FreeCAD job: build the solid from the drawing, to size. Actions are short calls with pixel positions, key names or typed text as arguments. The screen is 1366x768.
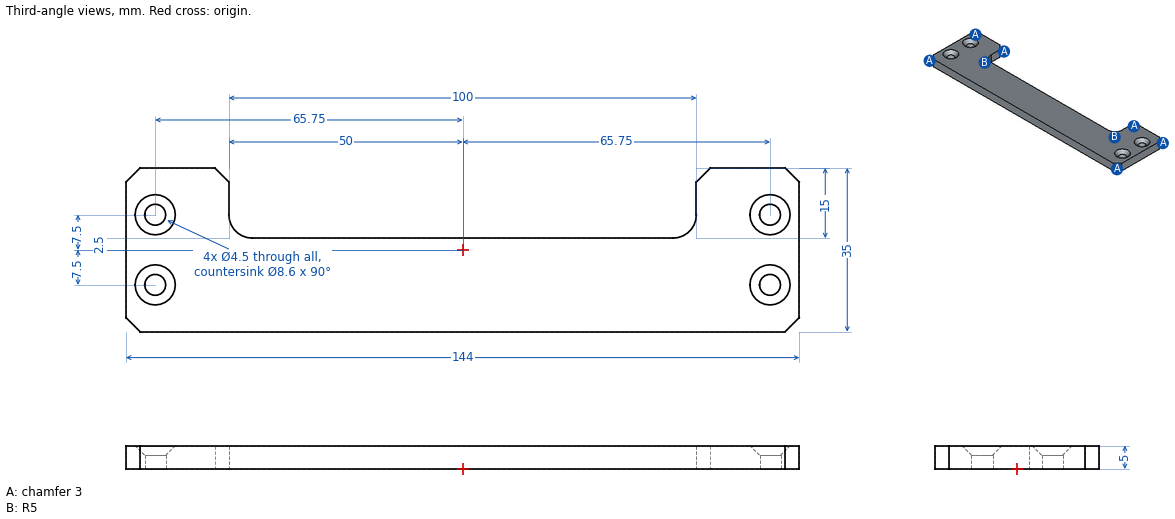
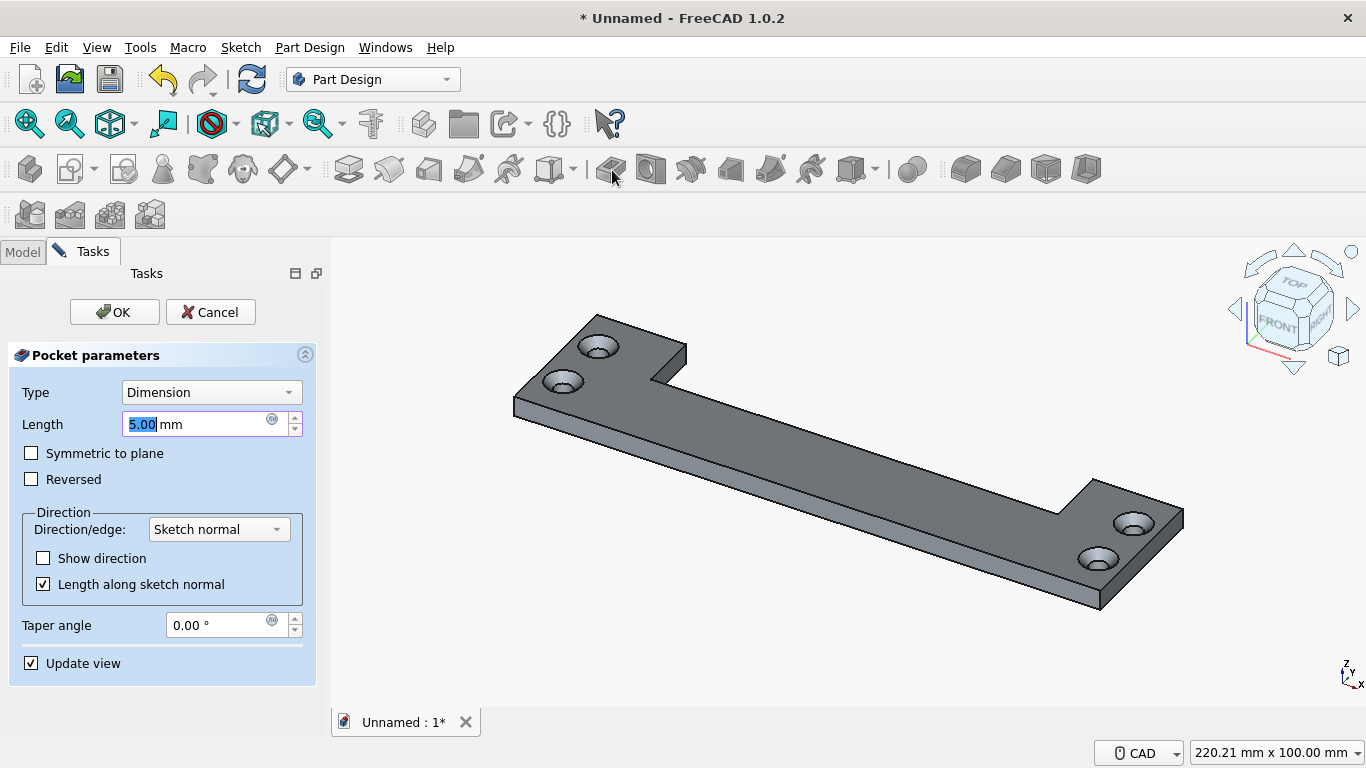
click(212, 392)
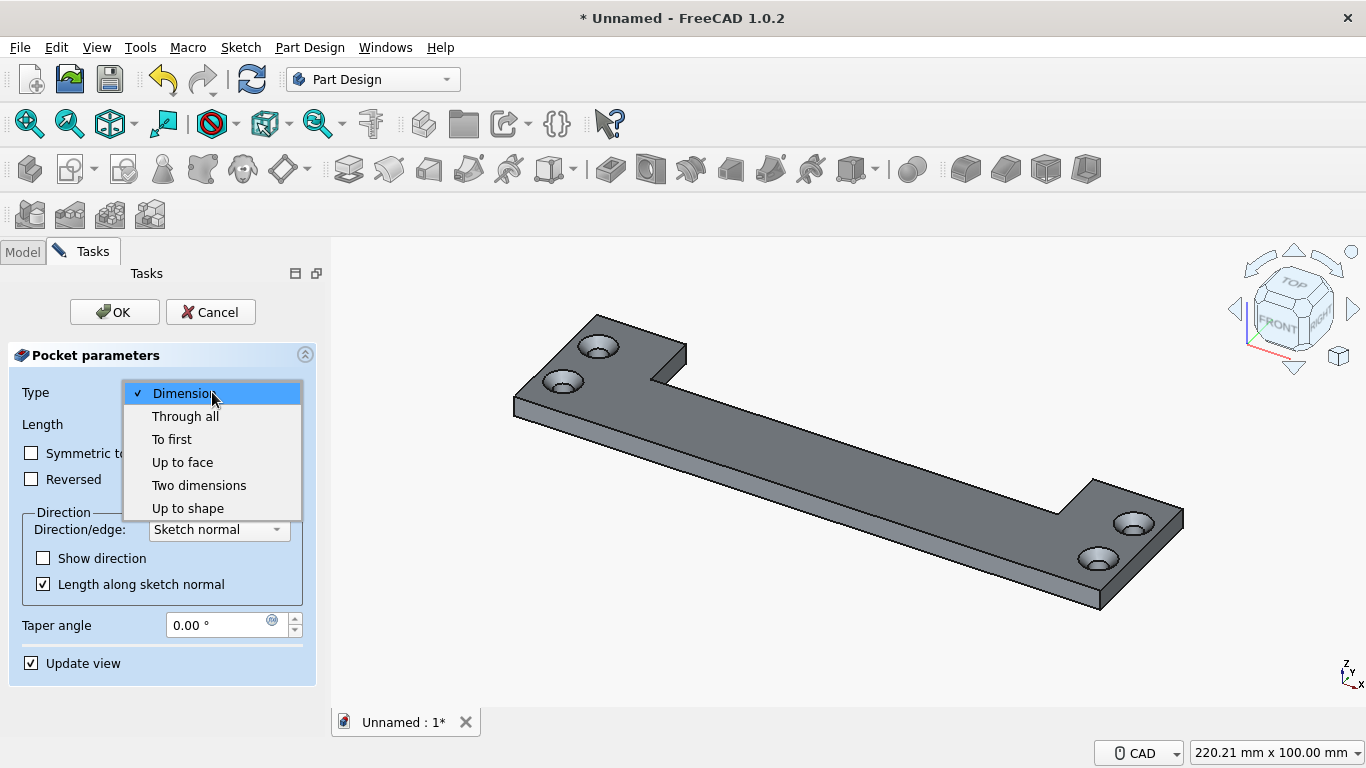
click(212, 416)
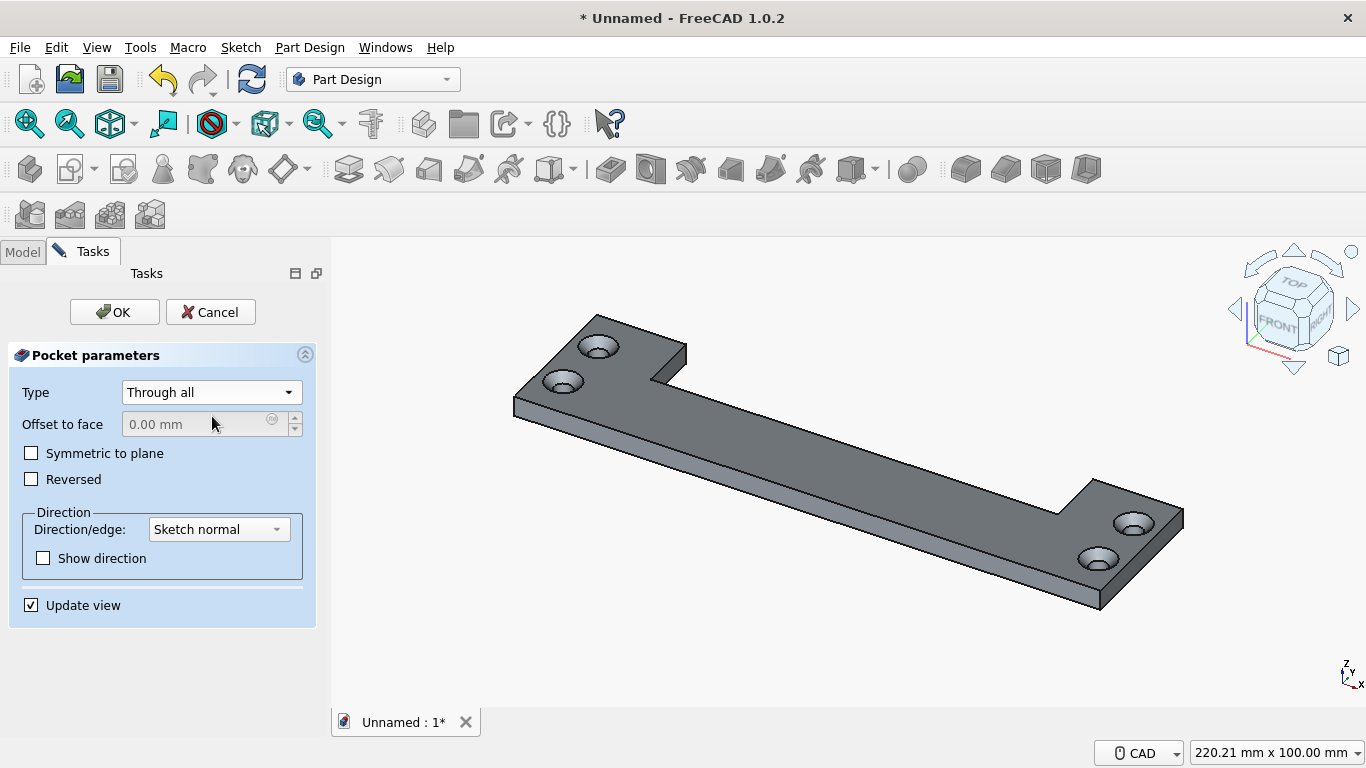
click(115, 312)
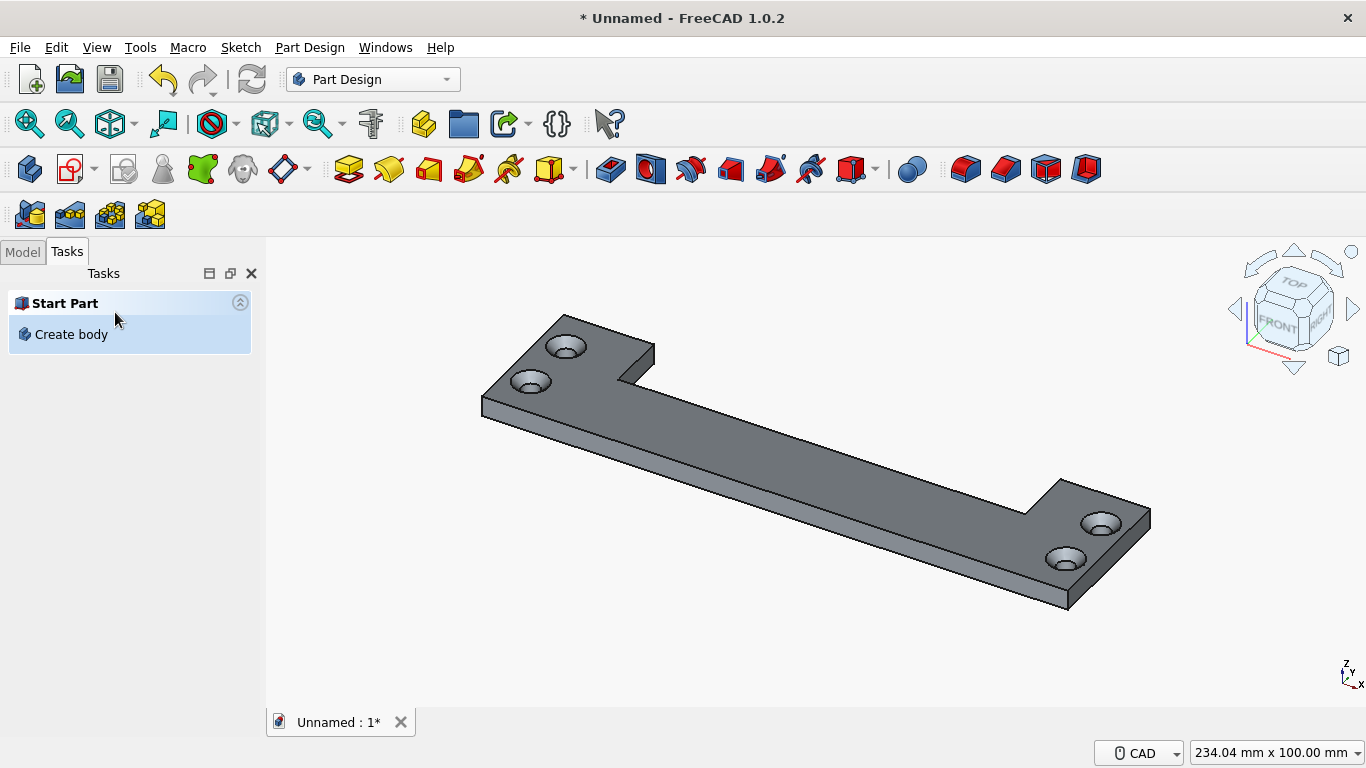
click(1068, 599)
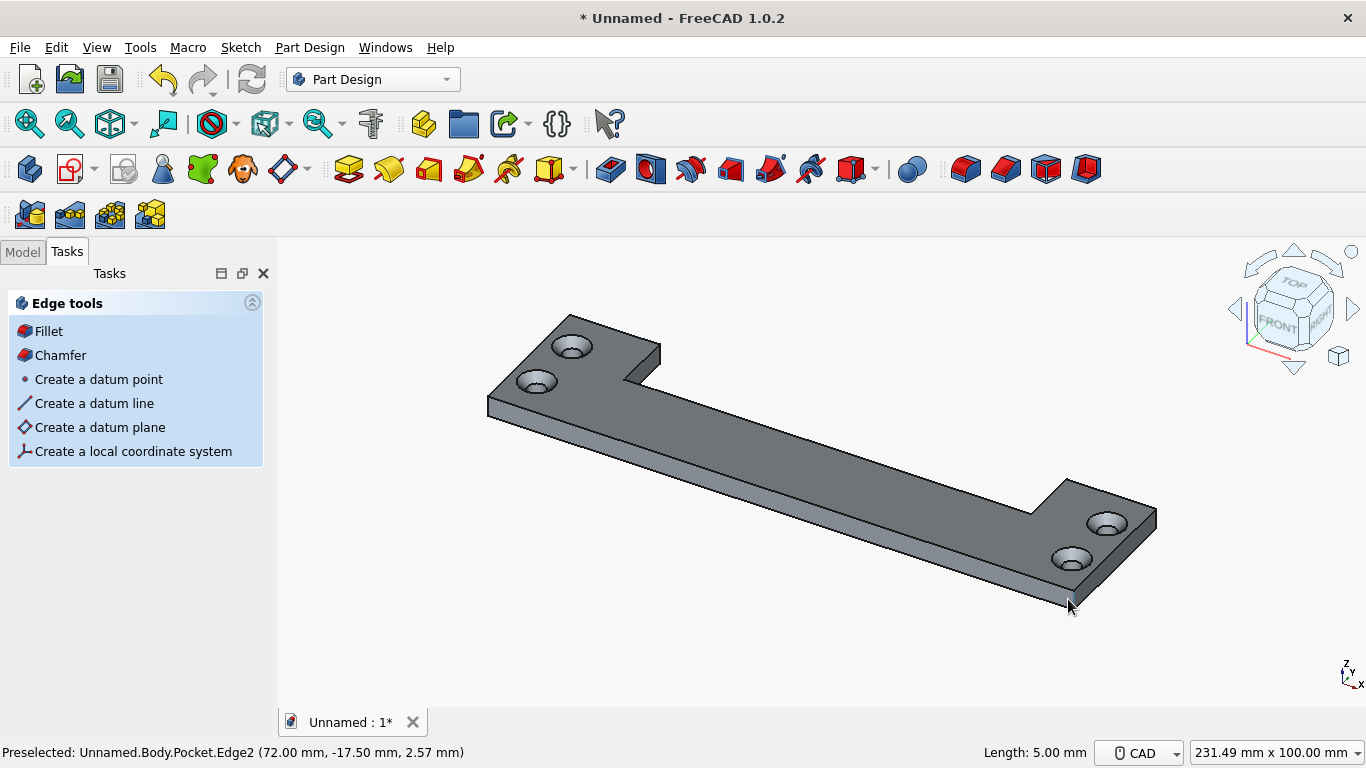
key(0)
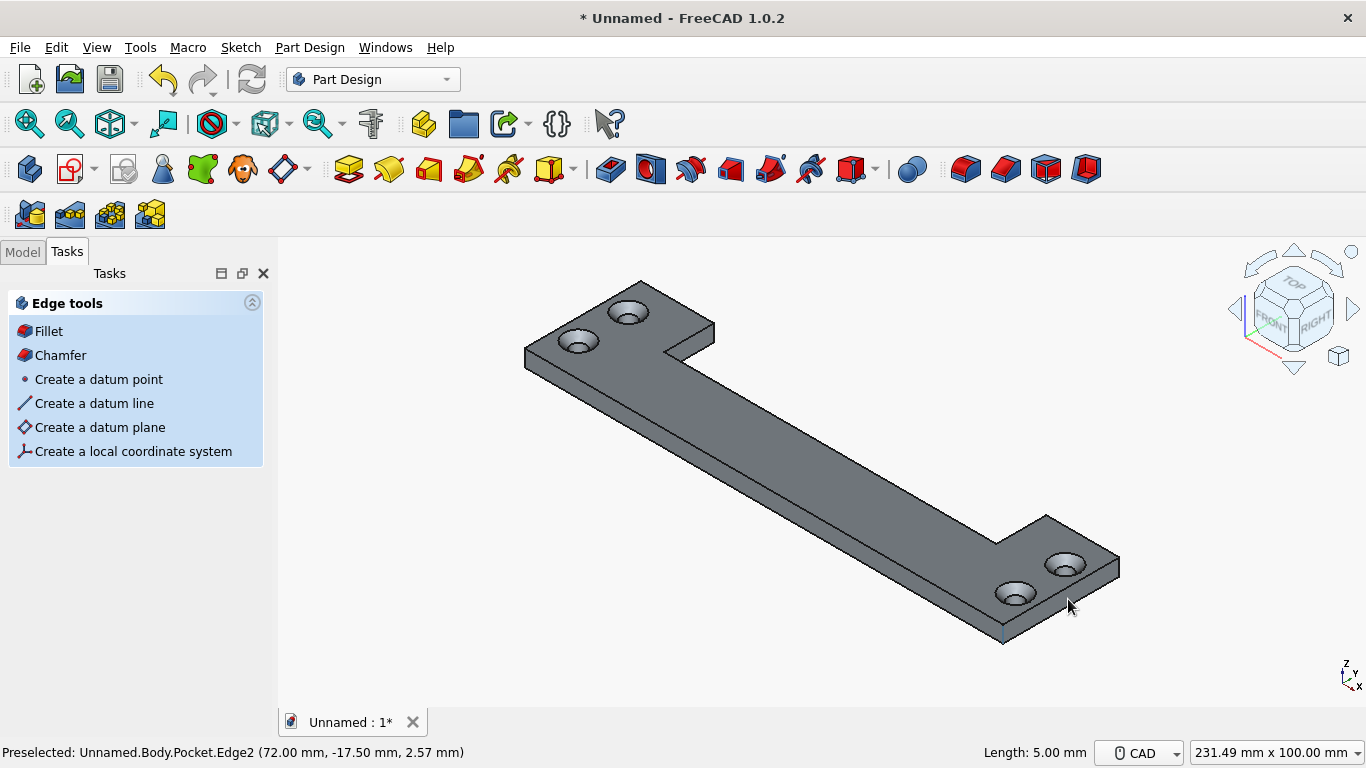
key(2)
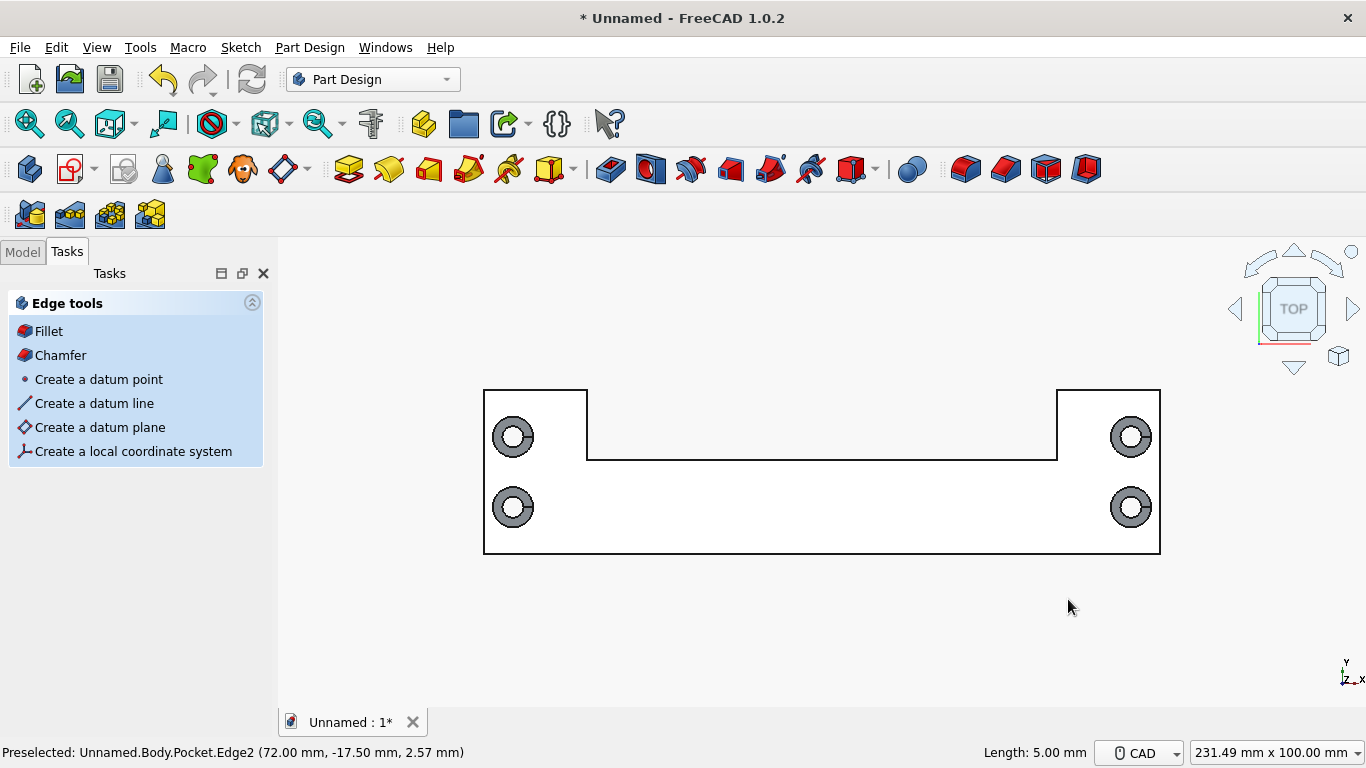
key(1)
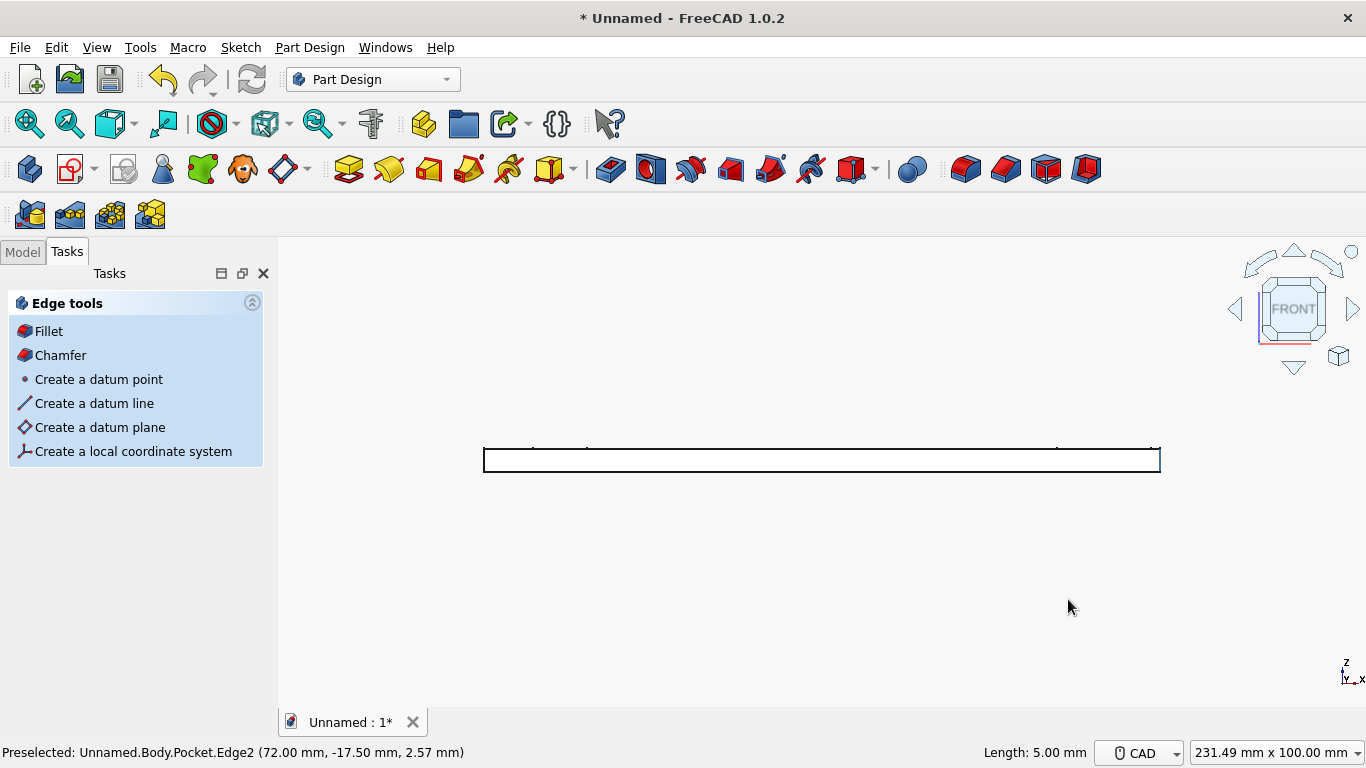
click(484, 459, ctrl)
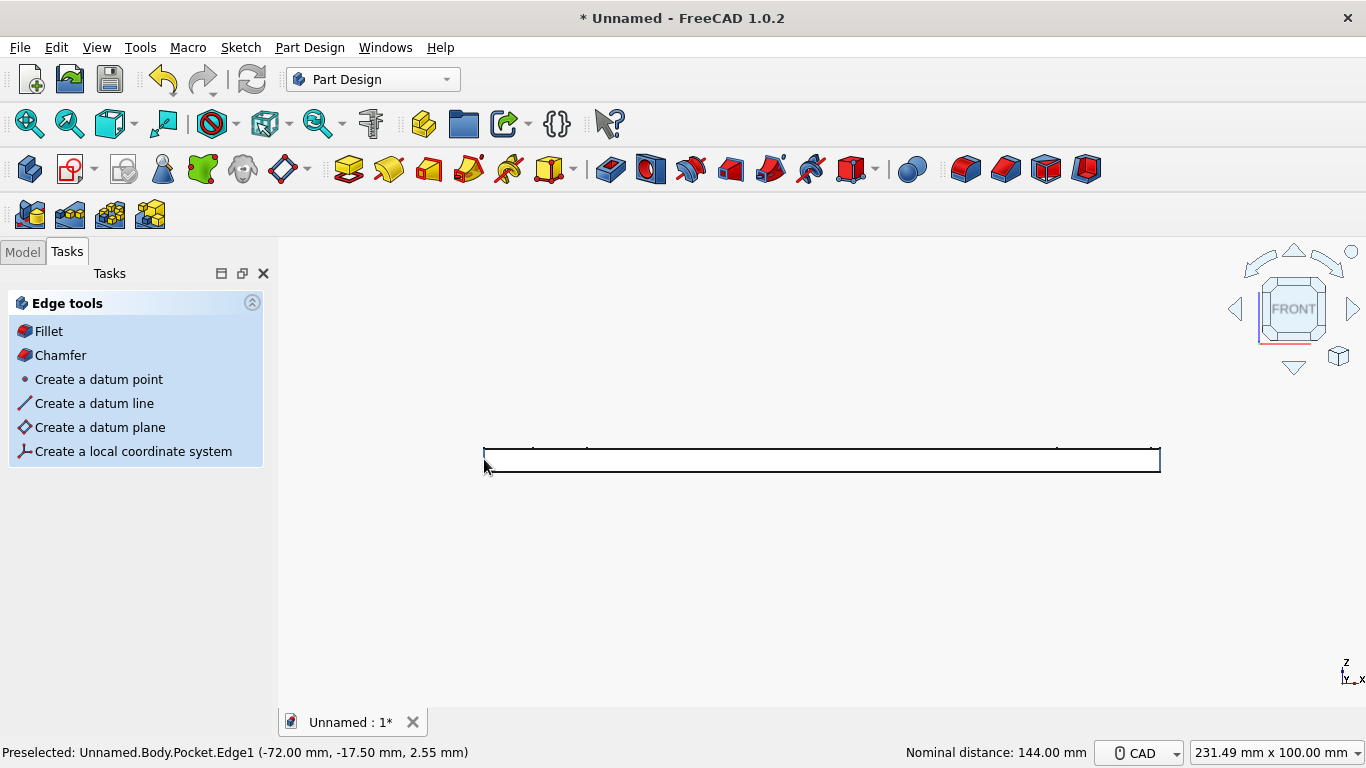
key(3)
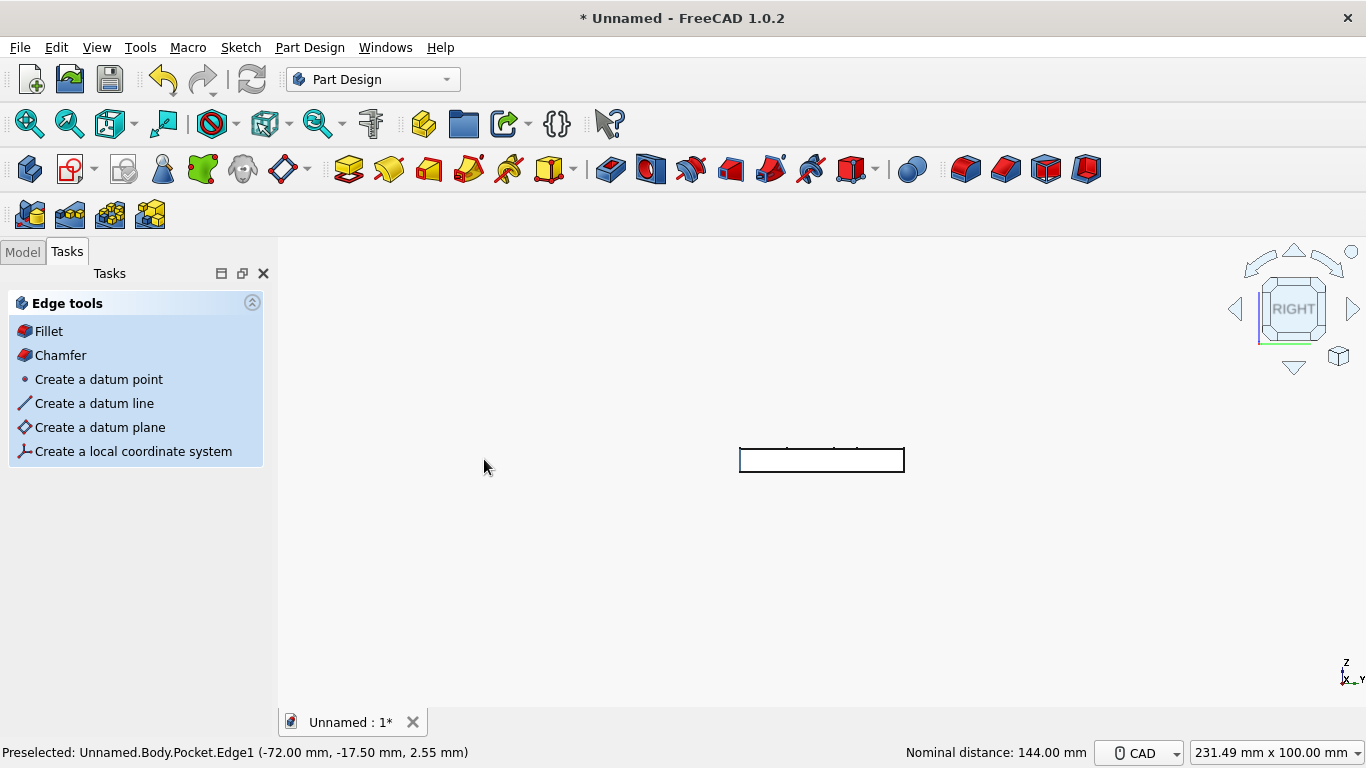
key(v)
key(f)